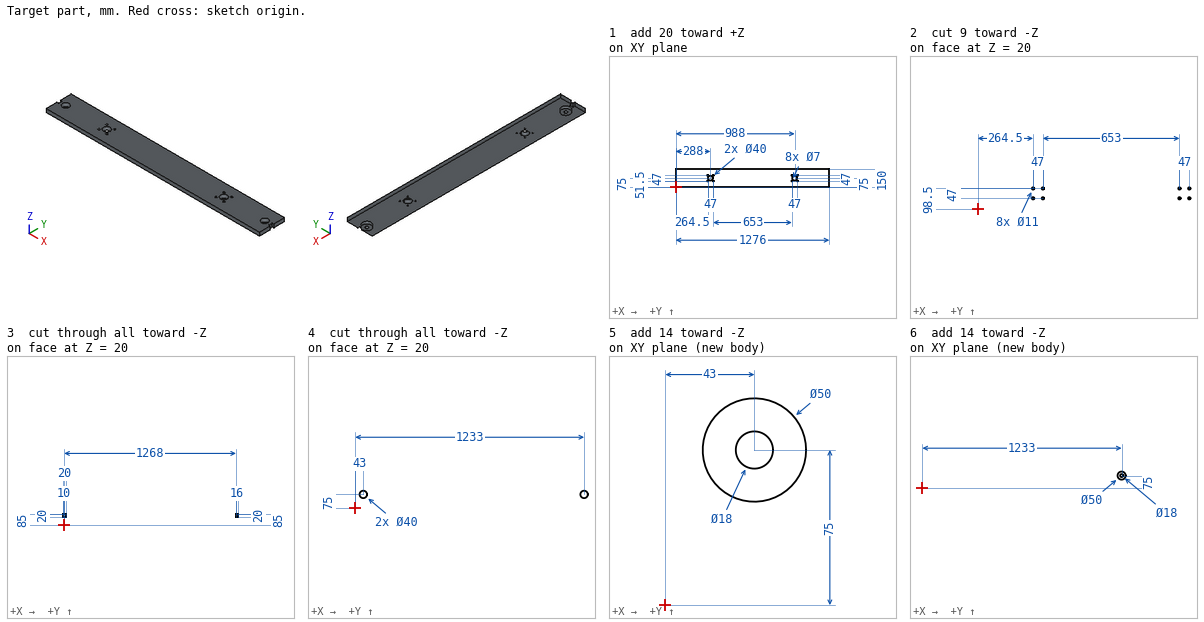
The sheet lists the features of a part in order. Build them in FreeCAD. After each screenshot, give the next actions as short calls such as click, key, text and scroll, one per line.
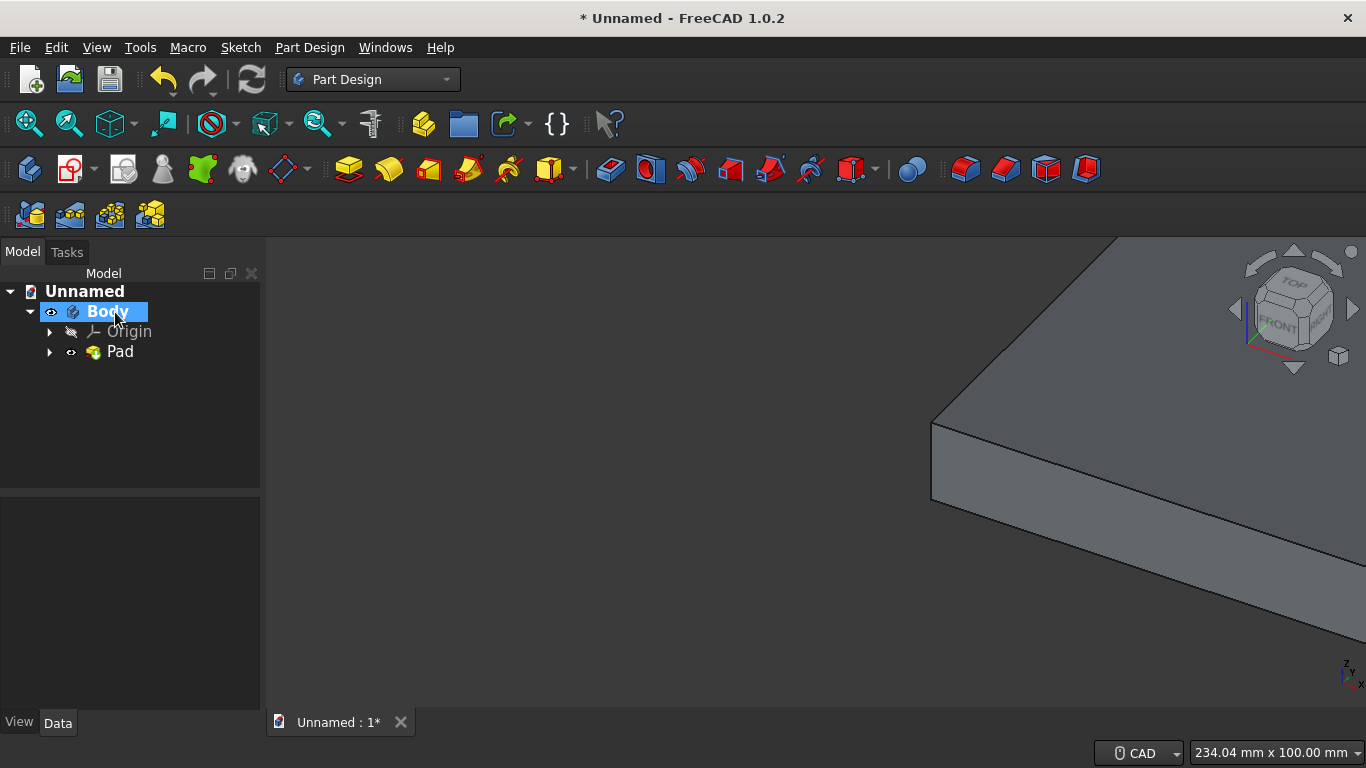
click(30, 124)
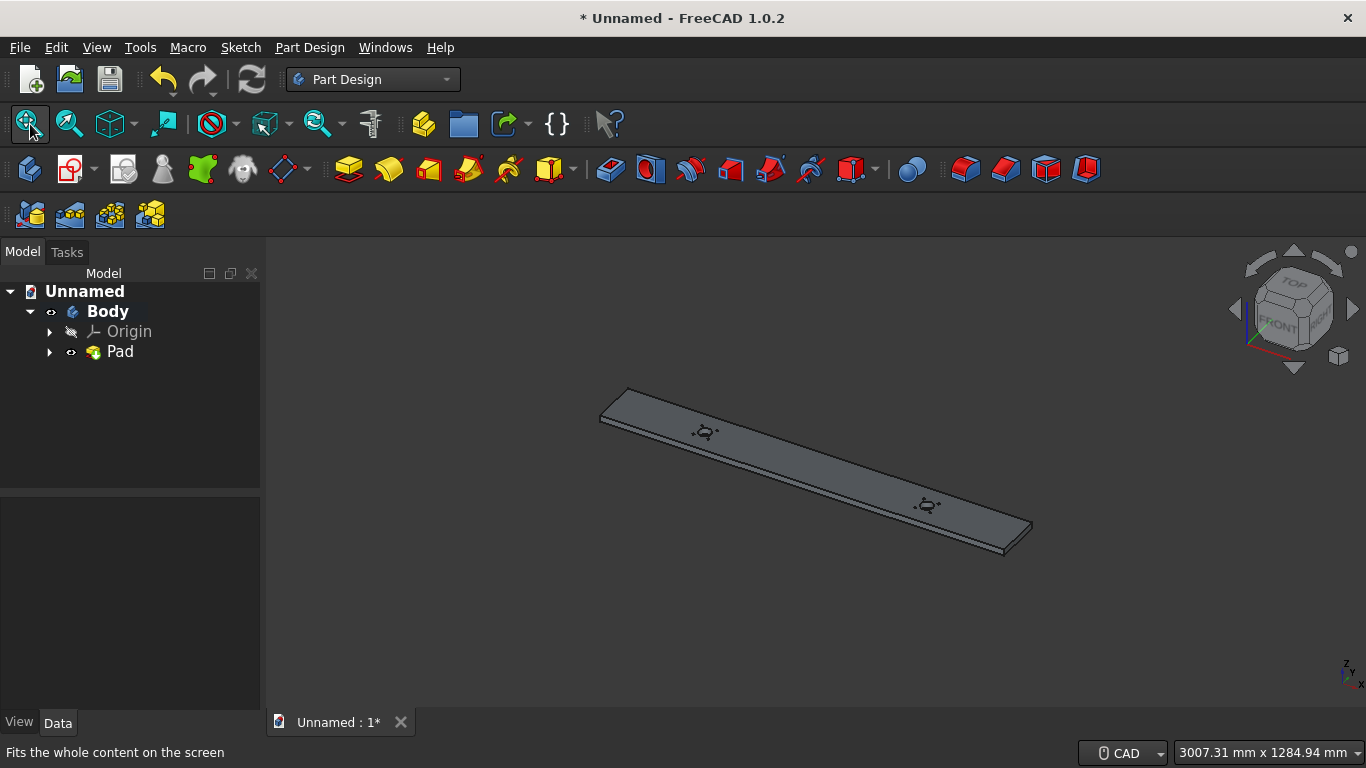
click(989, 525)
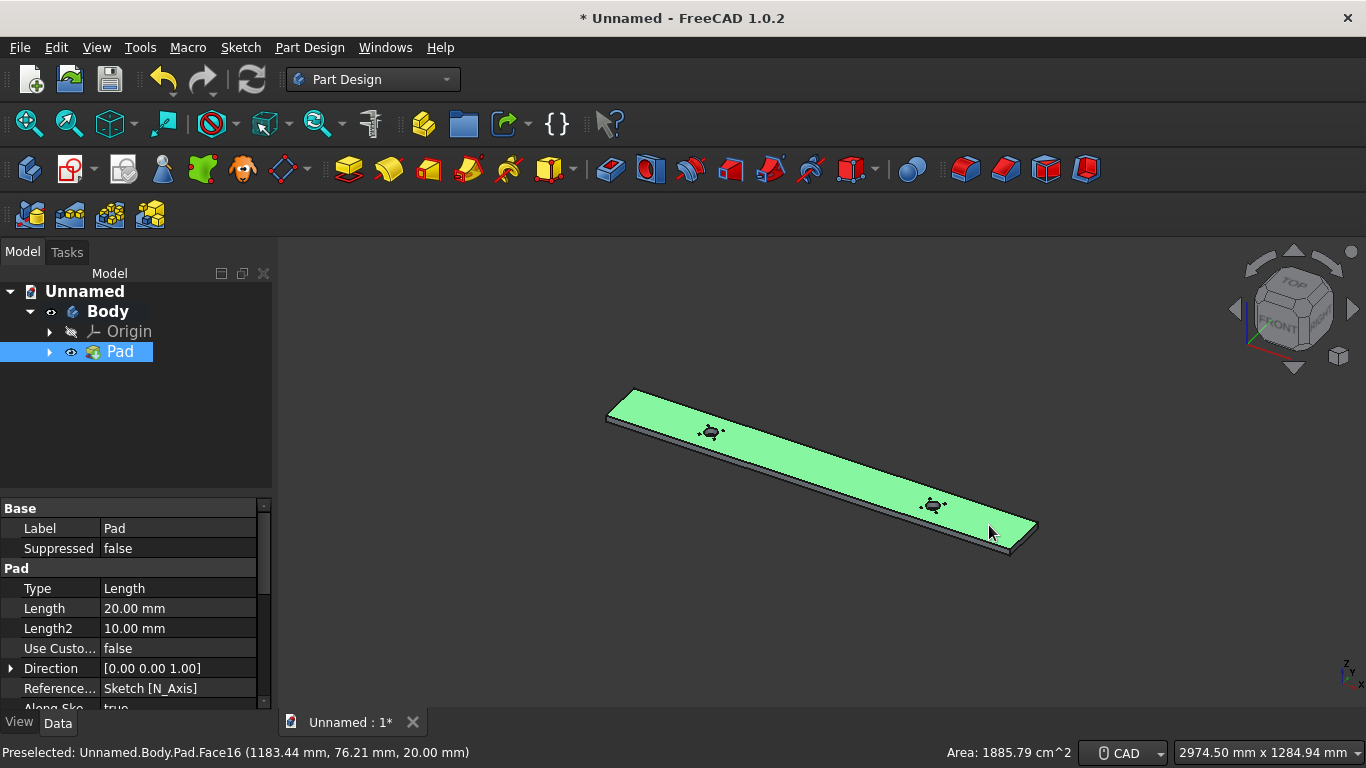
click(70, 170)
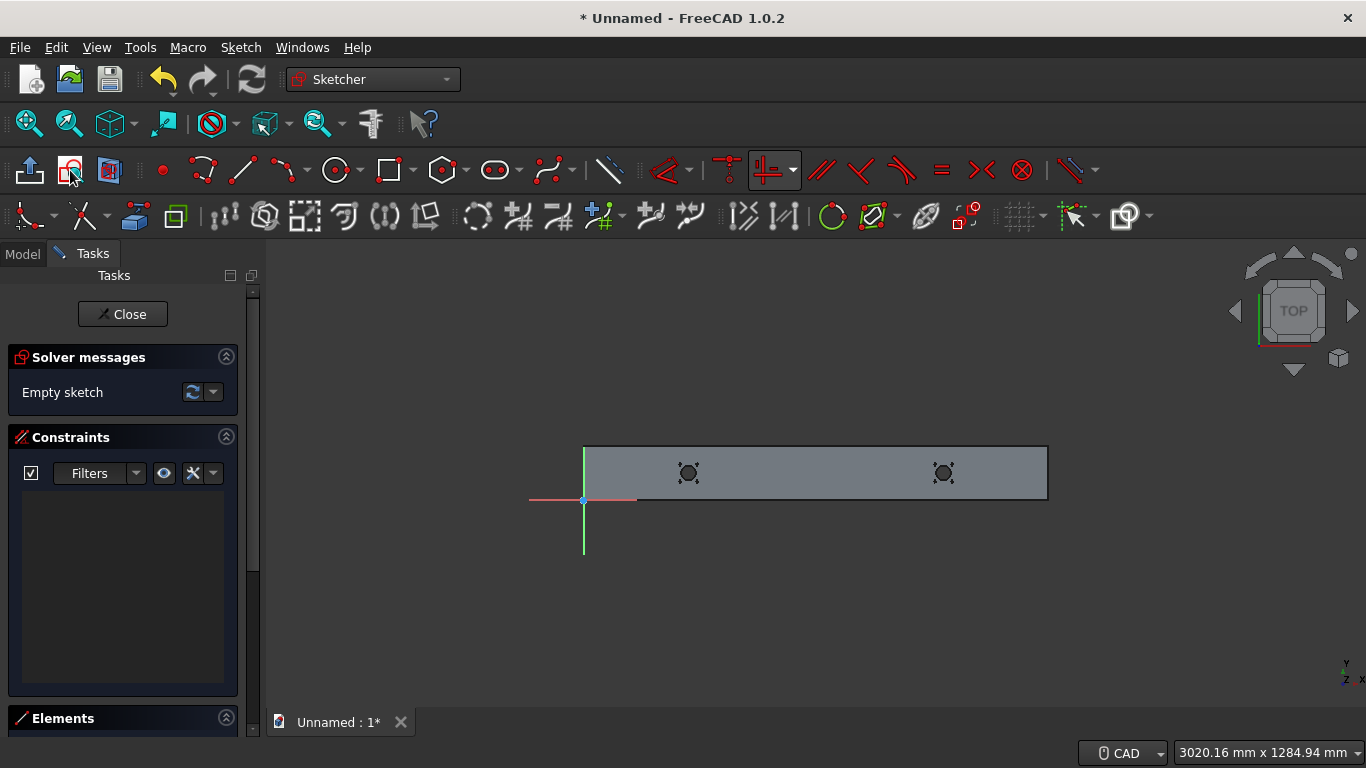
scroll(795, 492, up, 3)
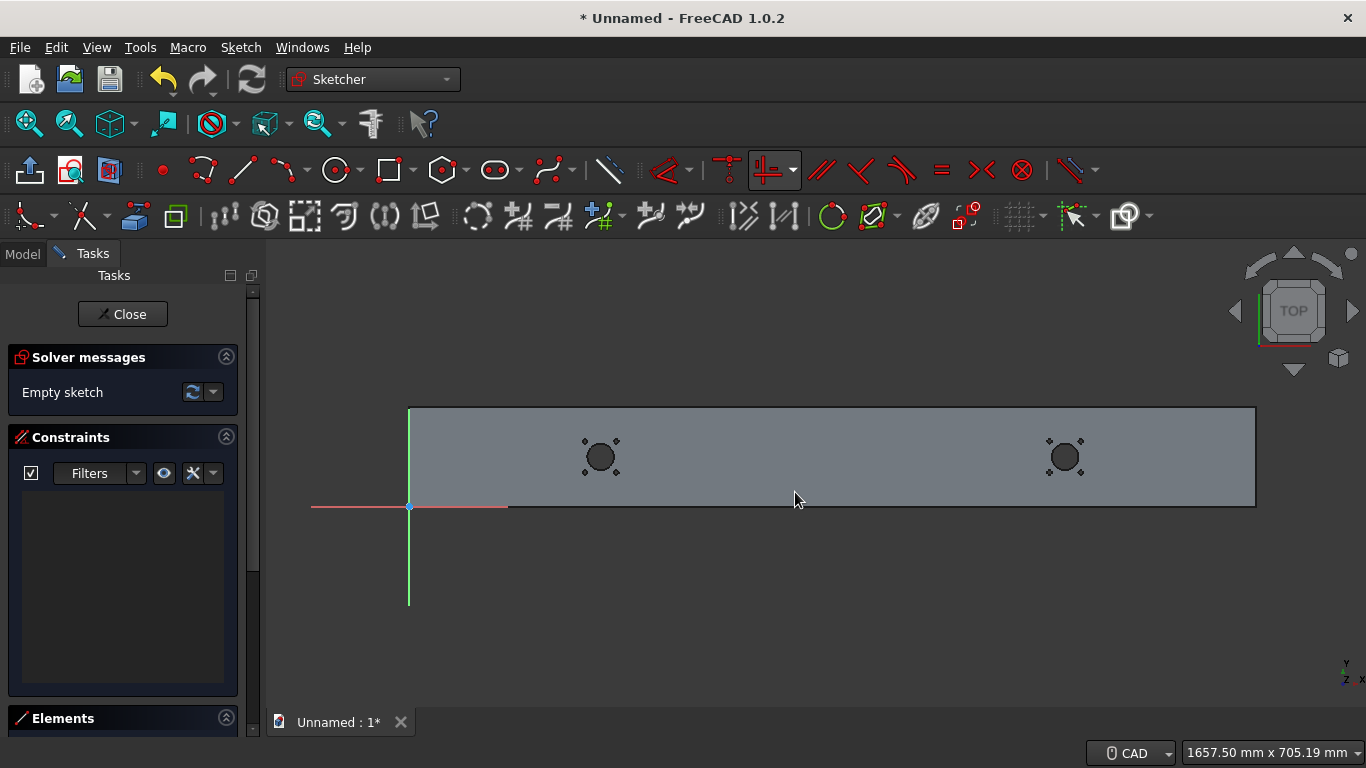
click(336, 170)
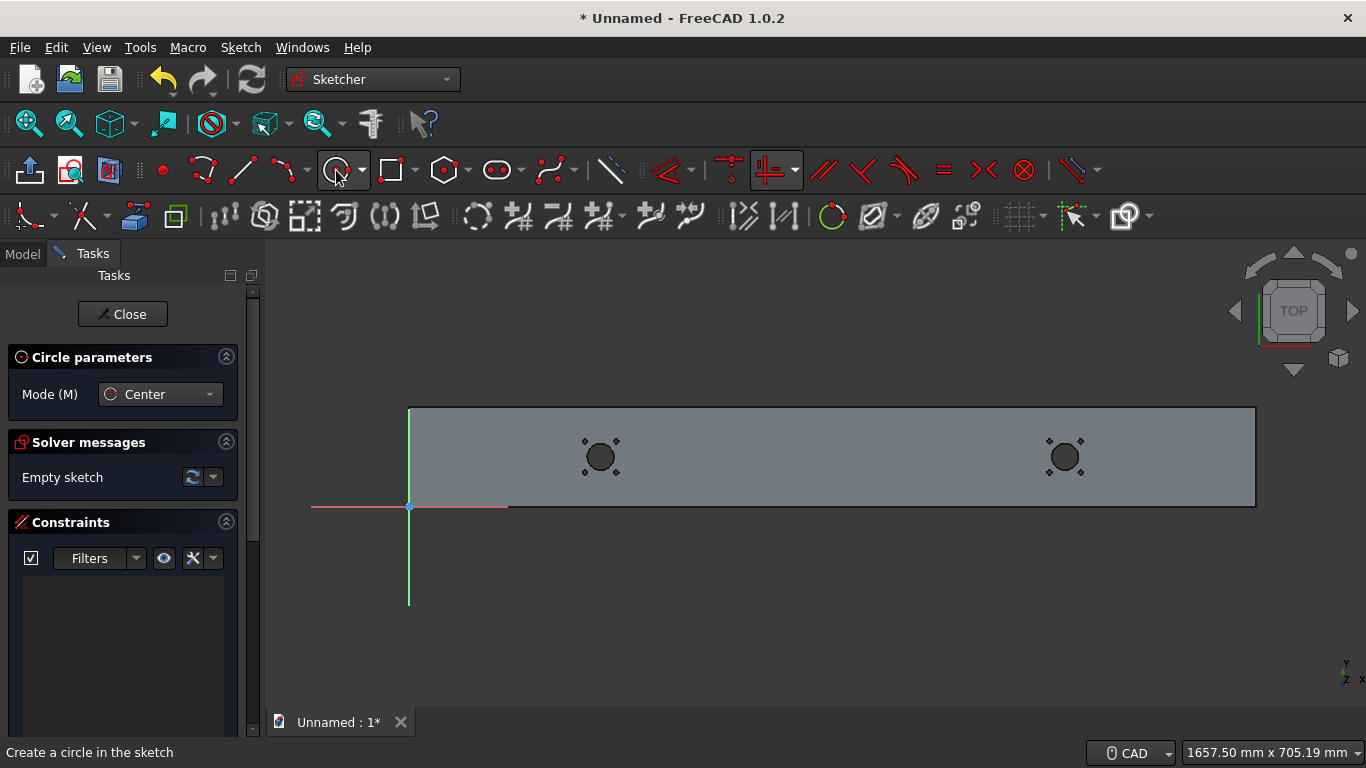
scroll(585, 441, up, 10)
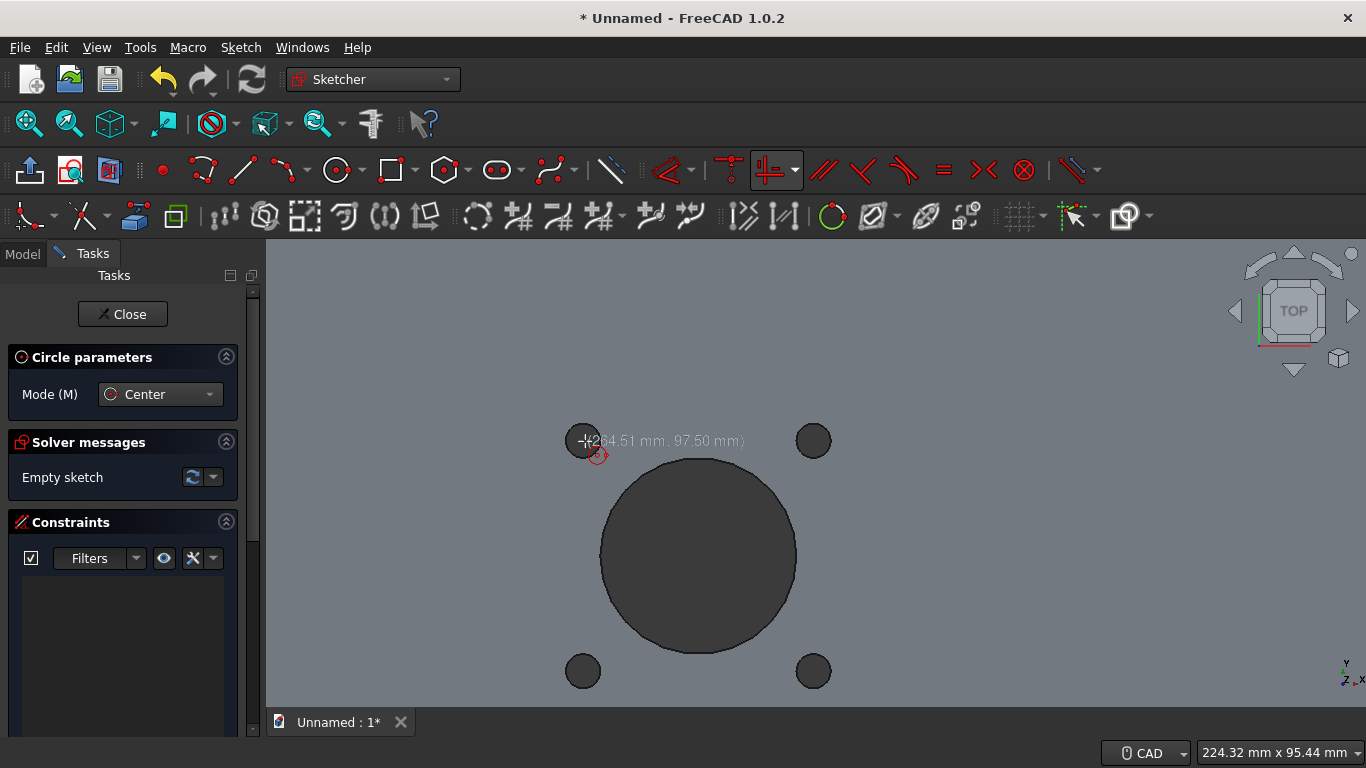
scroll(586, 442, down, 10)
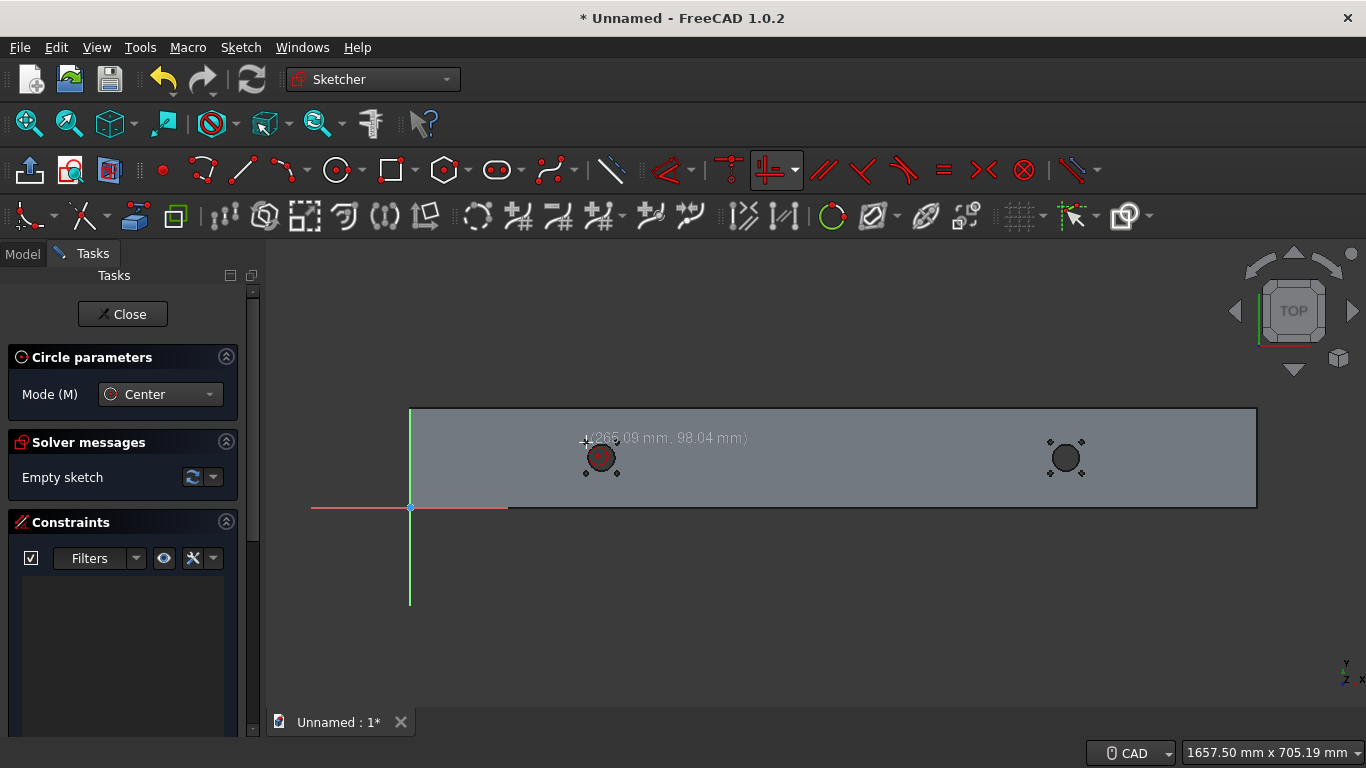
click(586, 442)
move(588, 440)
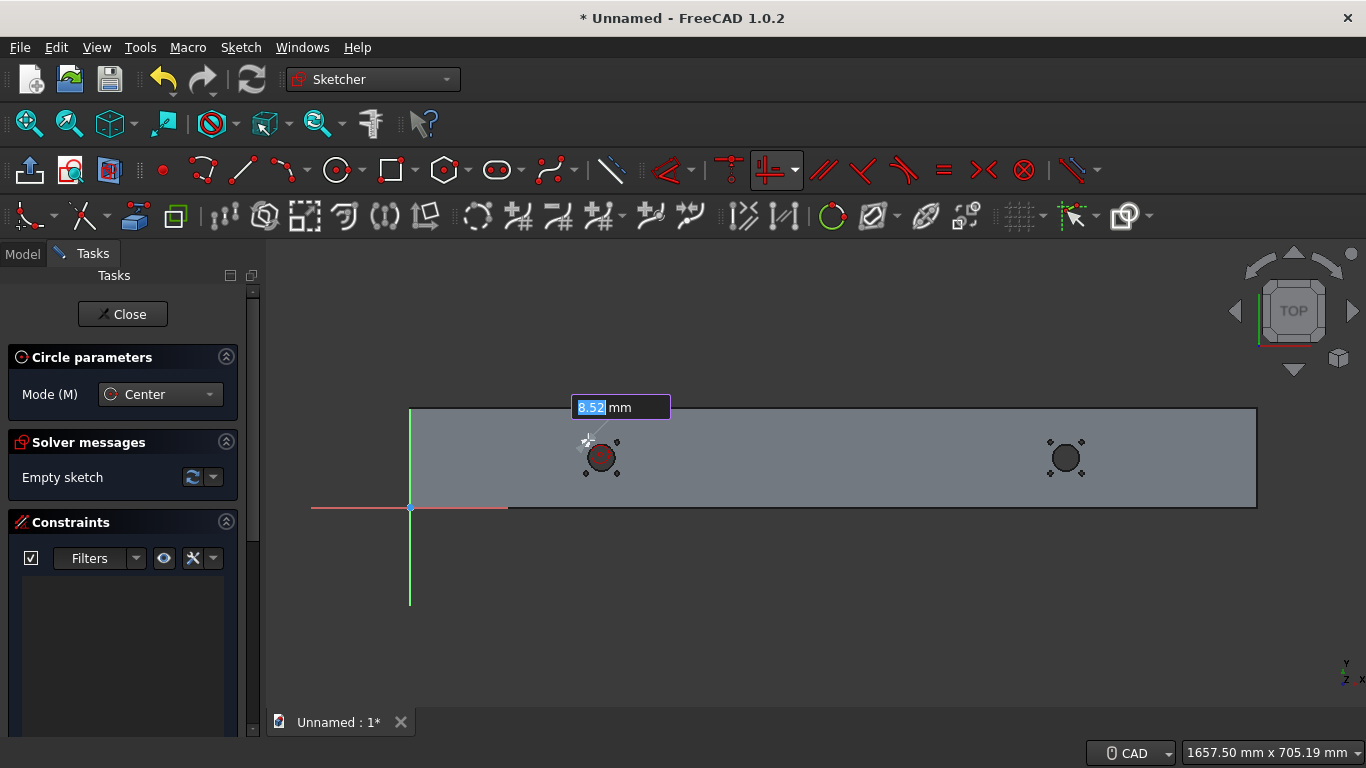
text(11)
key(Return)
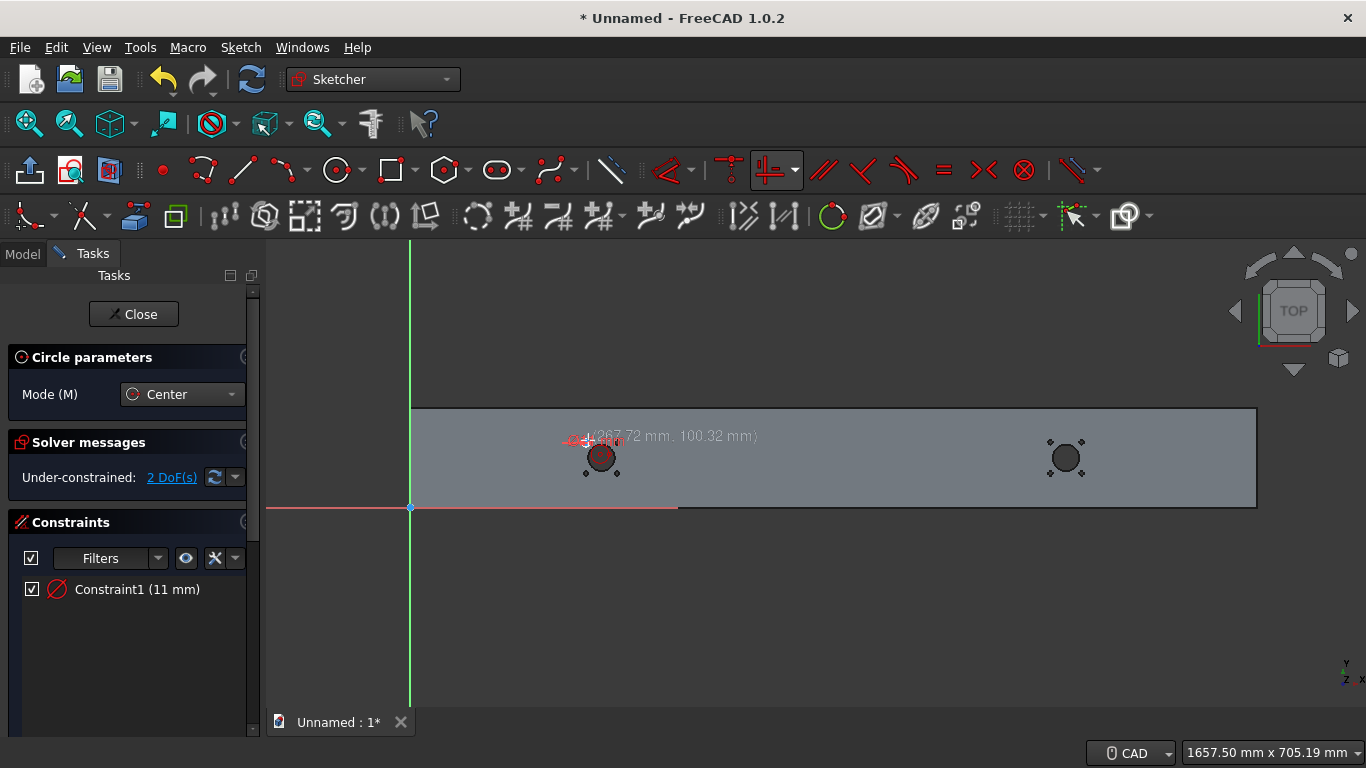
scroll(617, 442, up, 10)